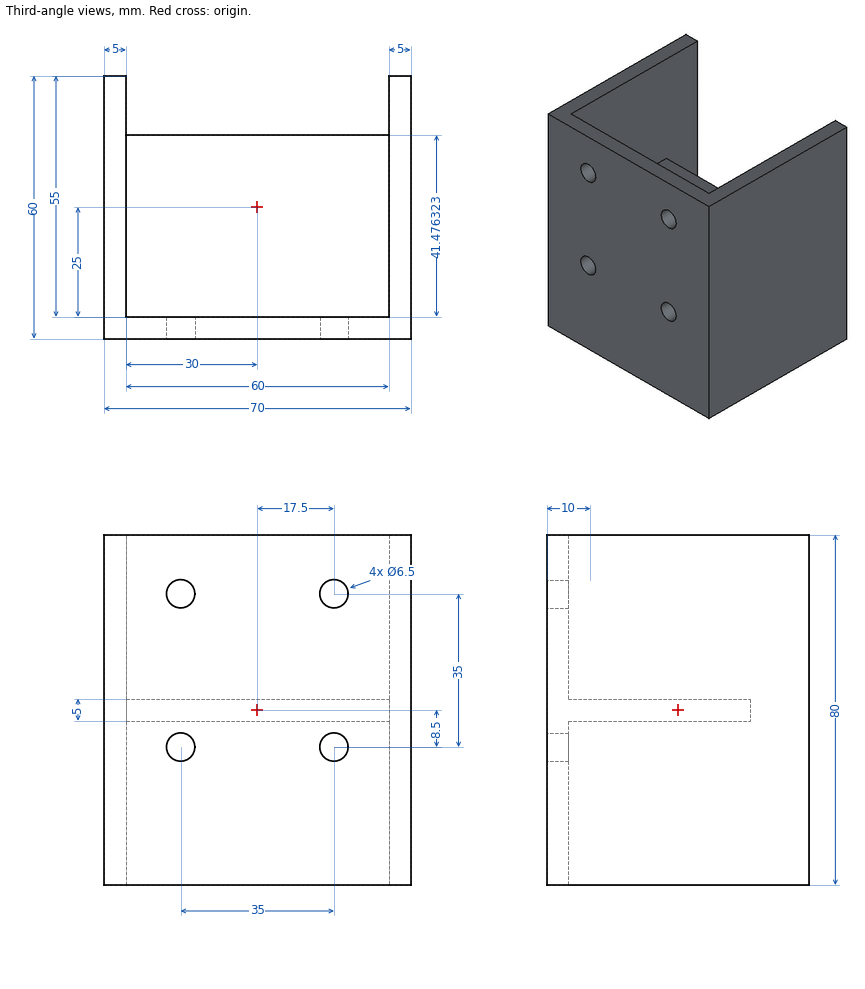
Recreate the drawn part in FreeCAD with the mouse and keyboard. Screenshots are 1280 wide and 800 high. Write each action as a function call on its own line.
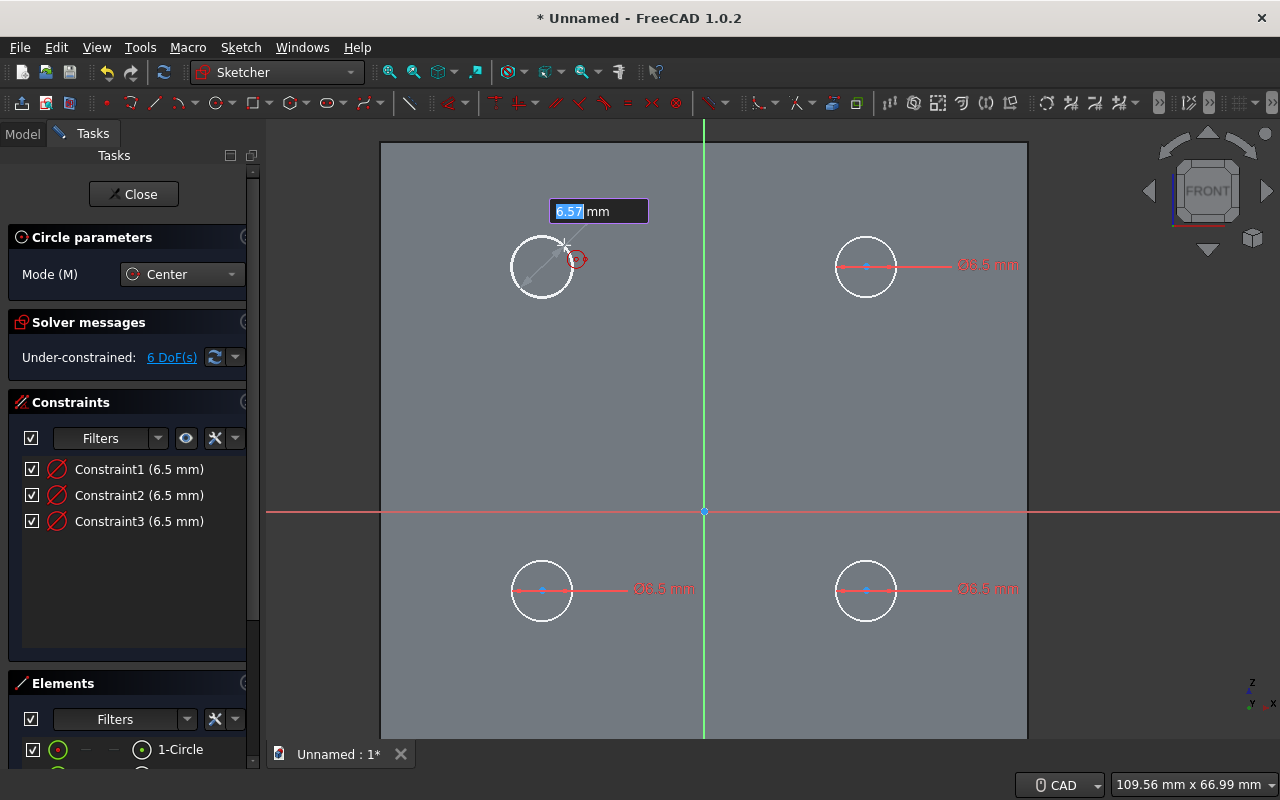
text(6.5)
key(Return)
key(Escape)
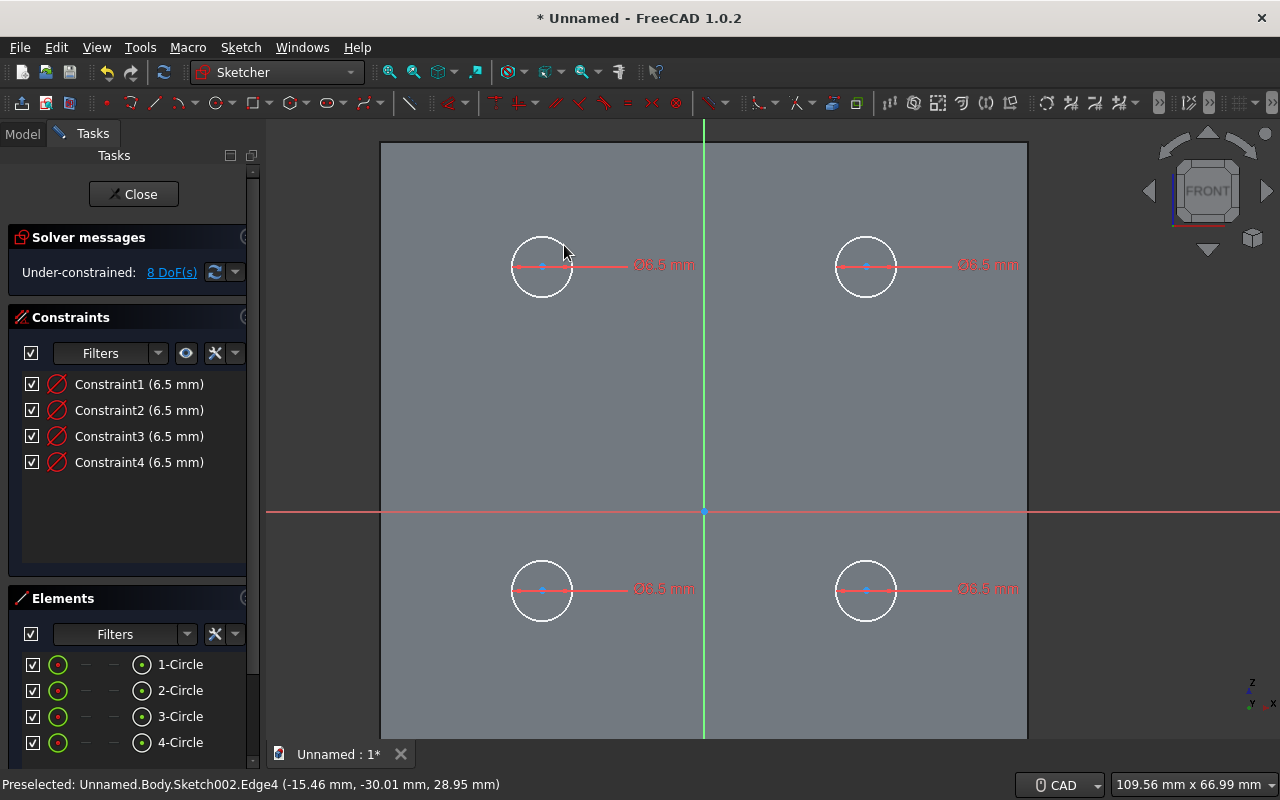
click(866, 267)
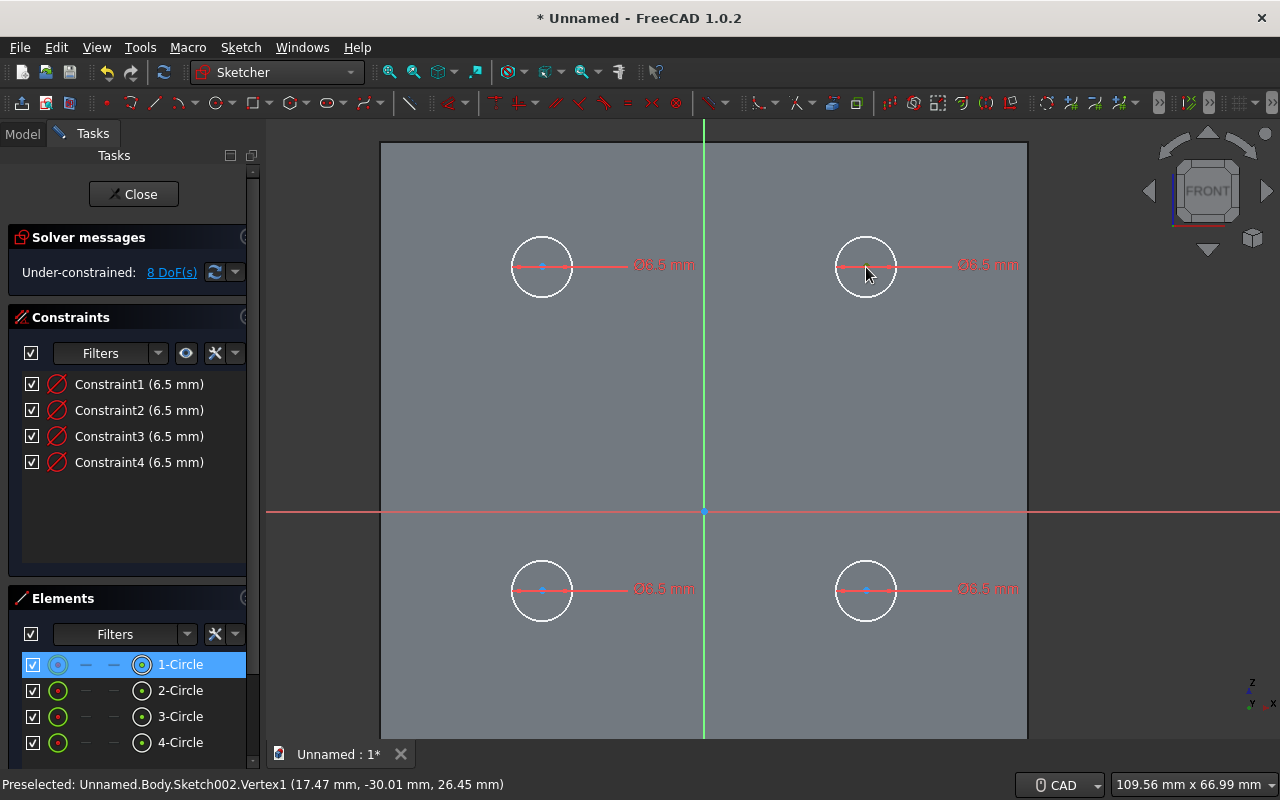
click(866, 591)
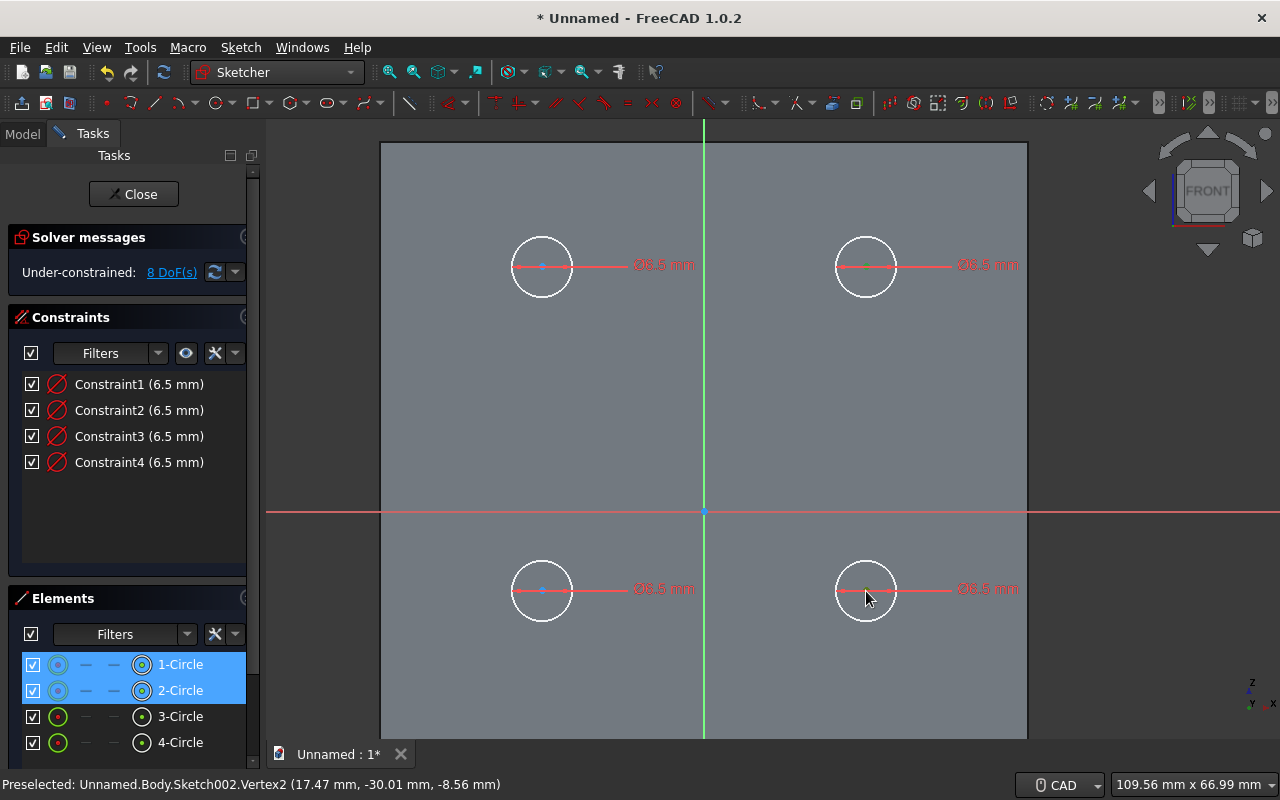
key(v)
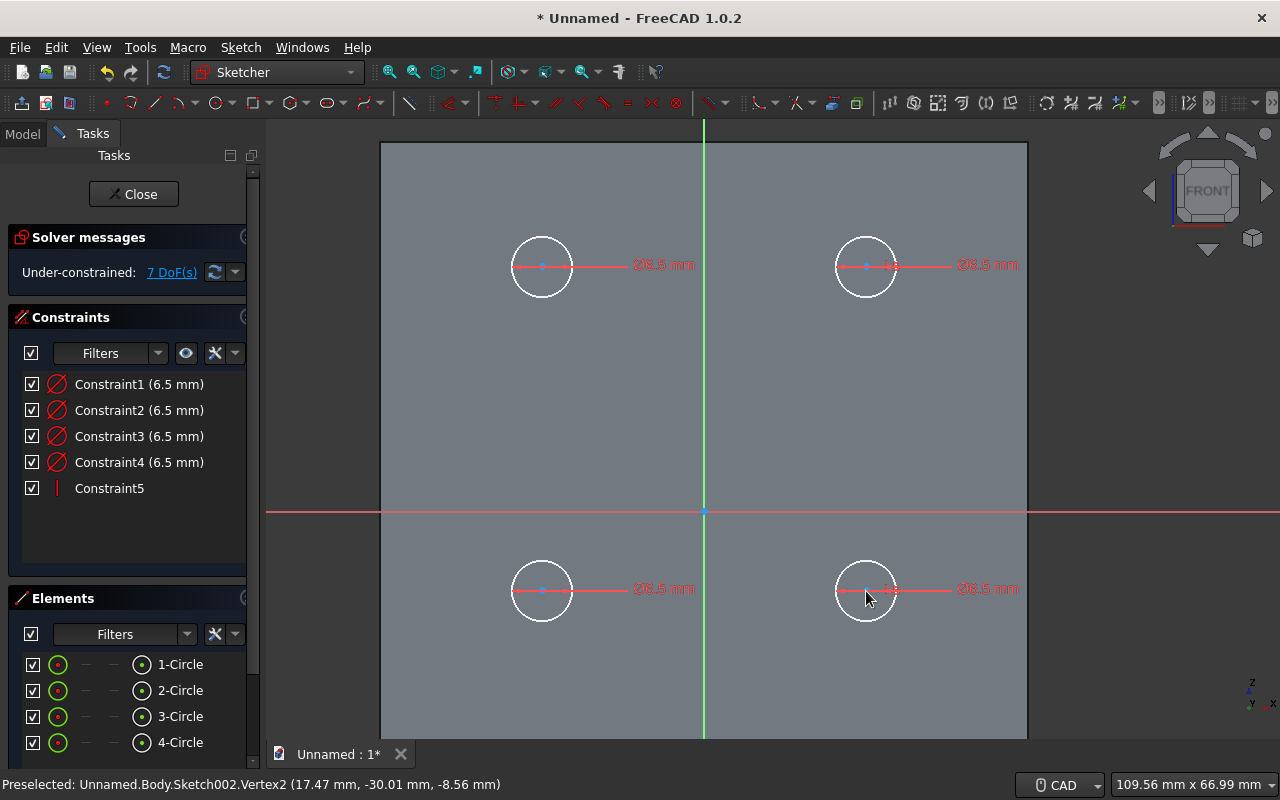
click(866, 591)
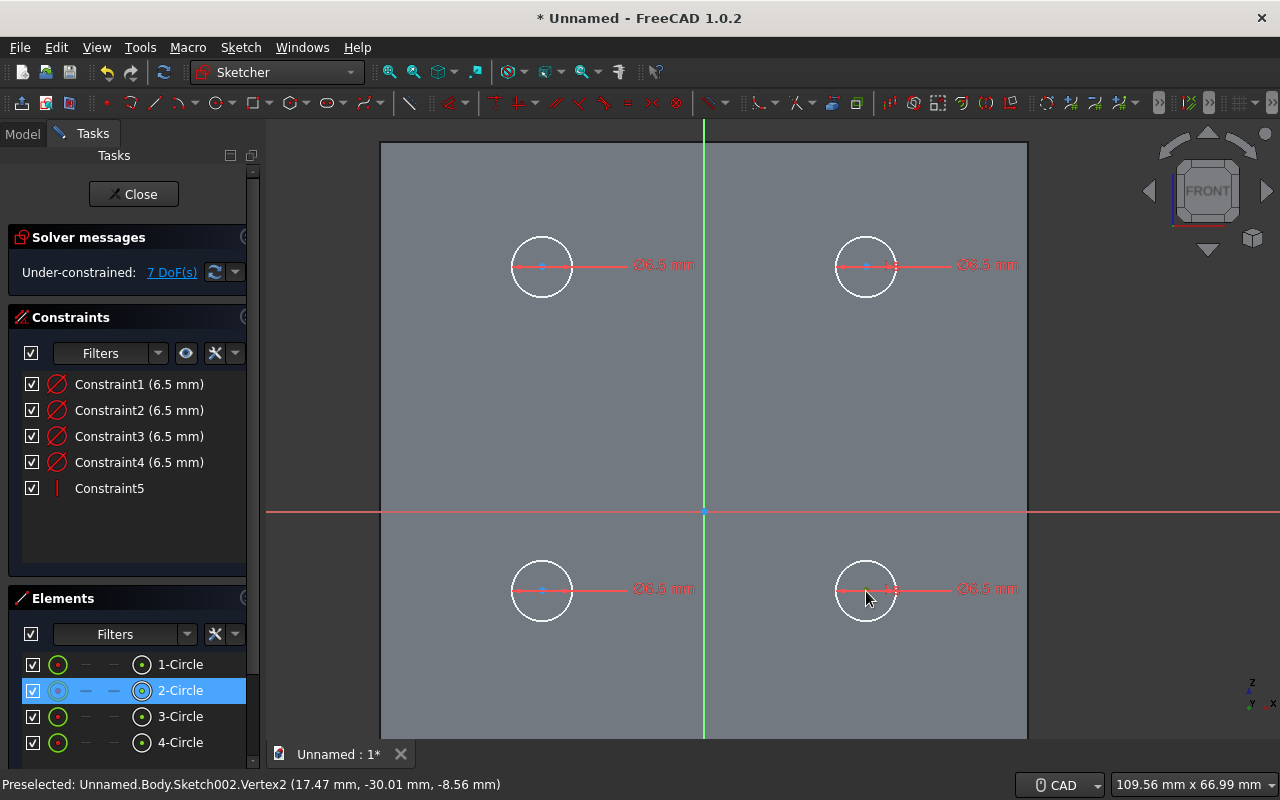
click(542, 591)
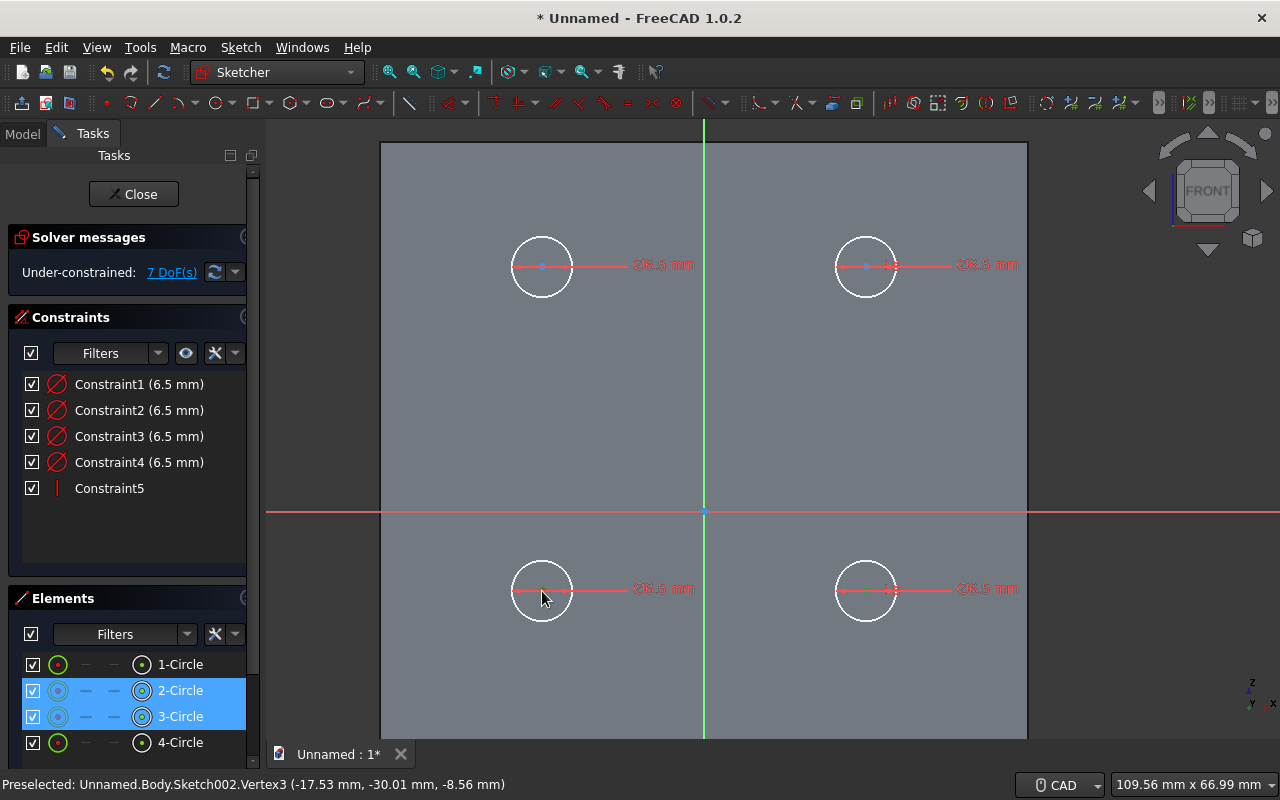
key(h)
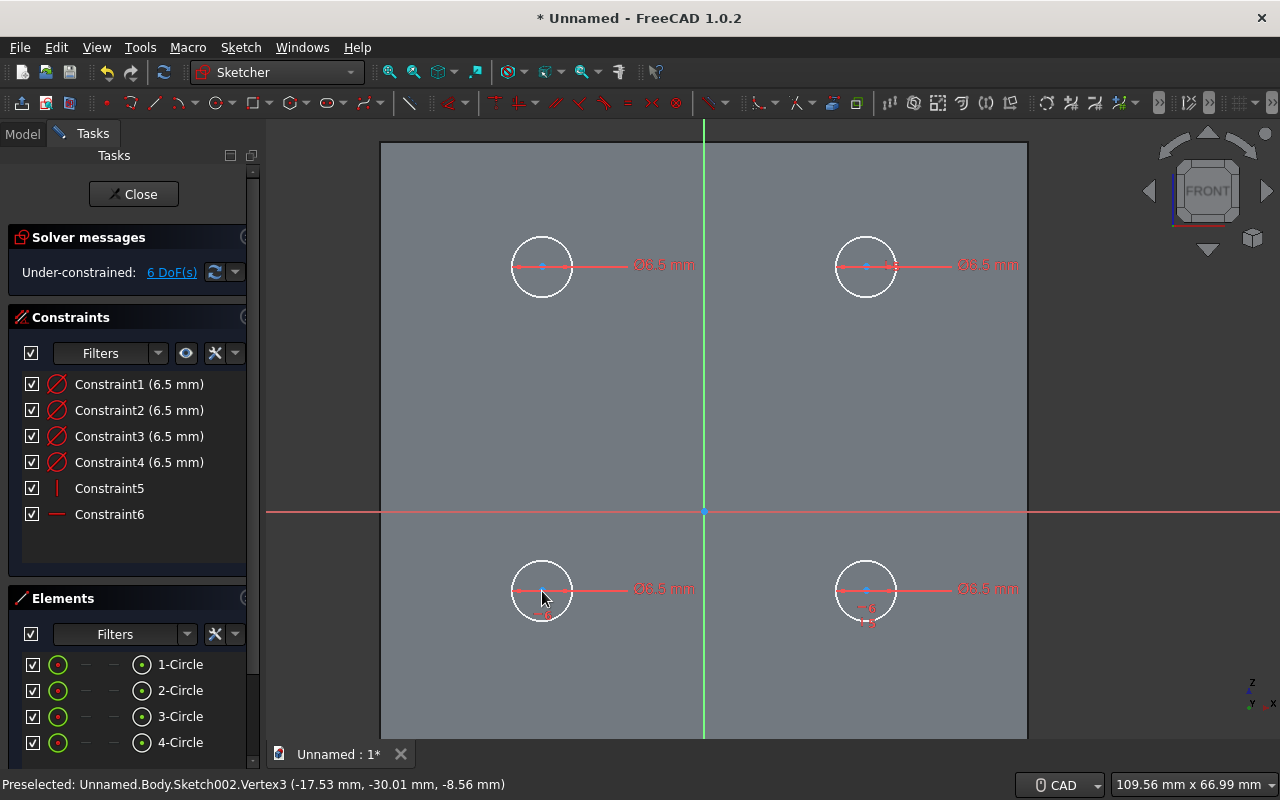
click(542, 591)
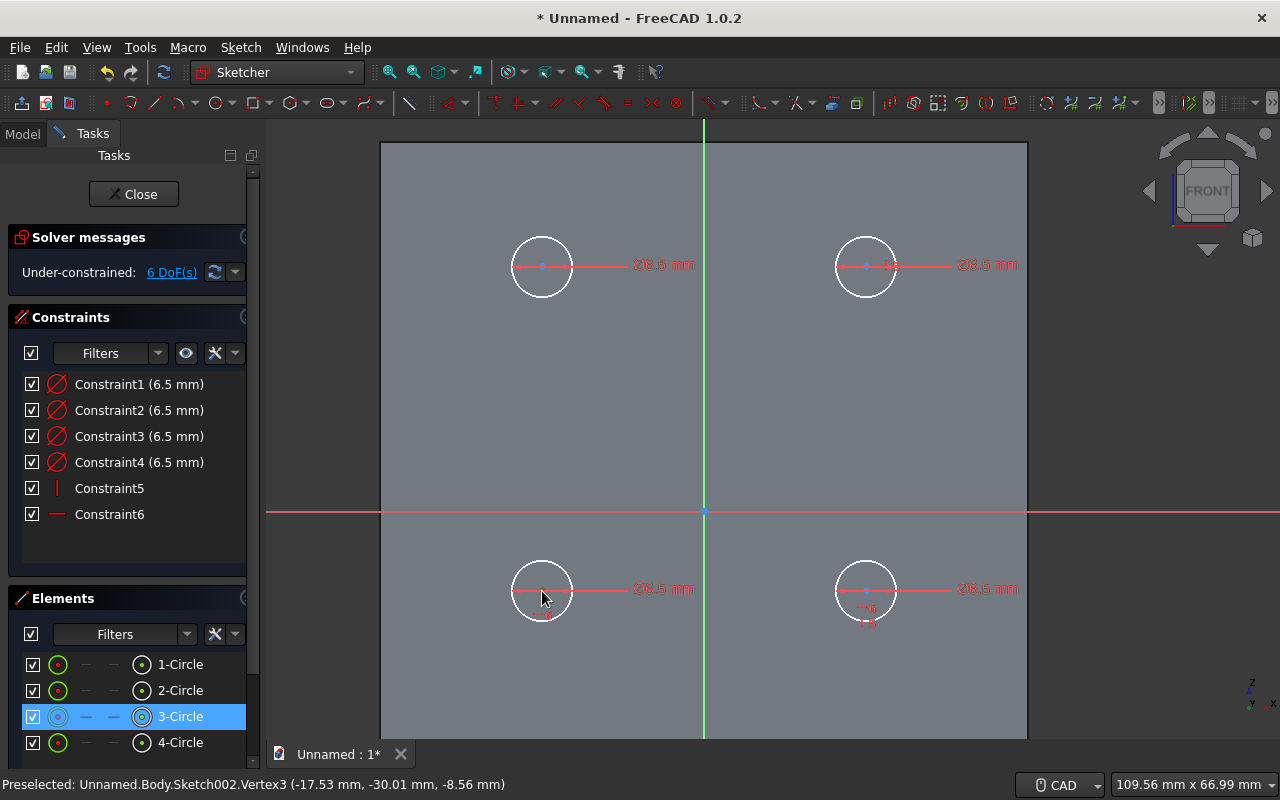
click(542, 267)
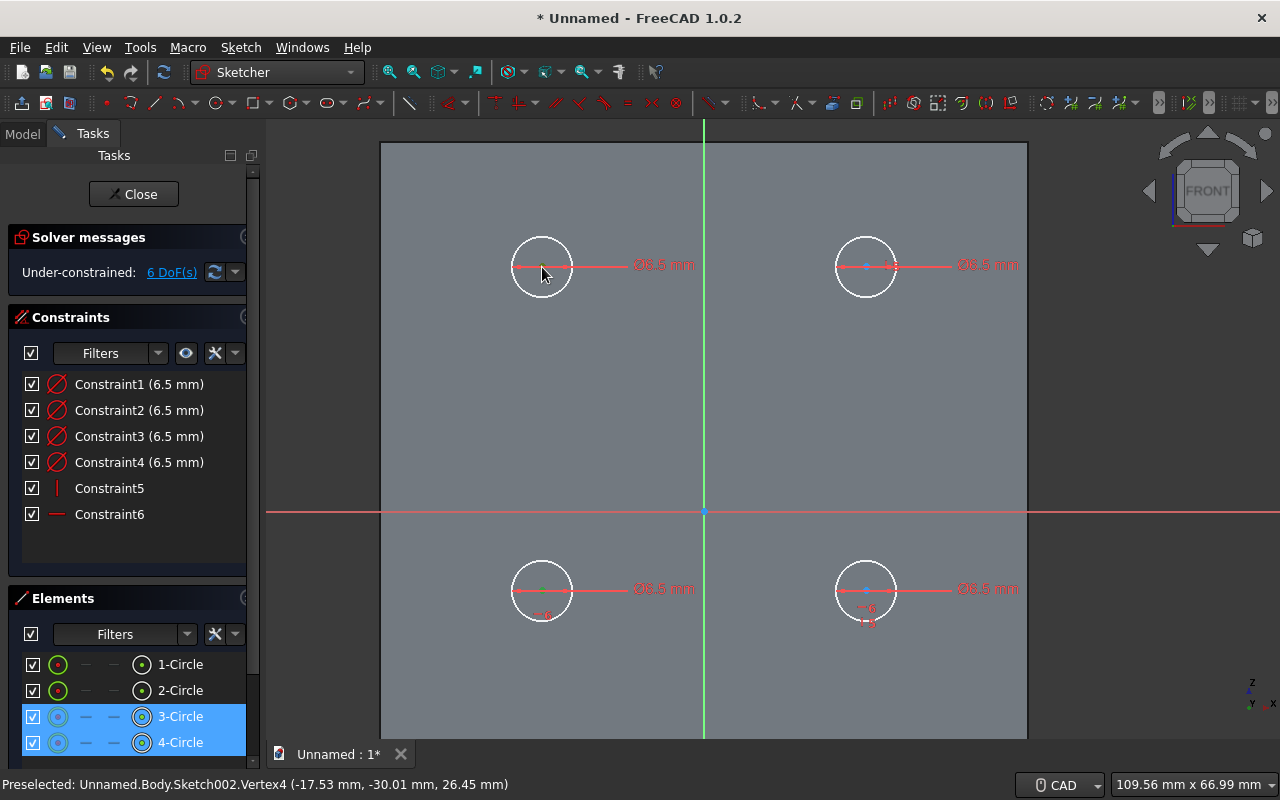
click(538, 104)